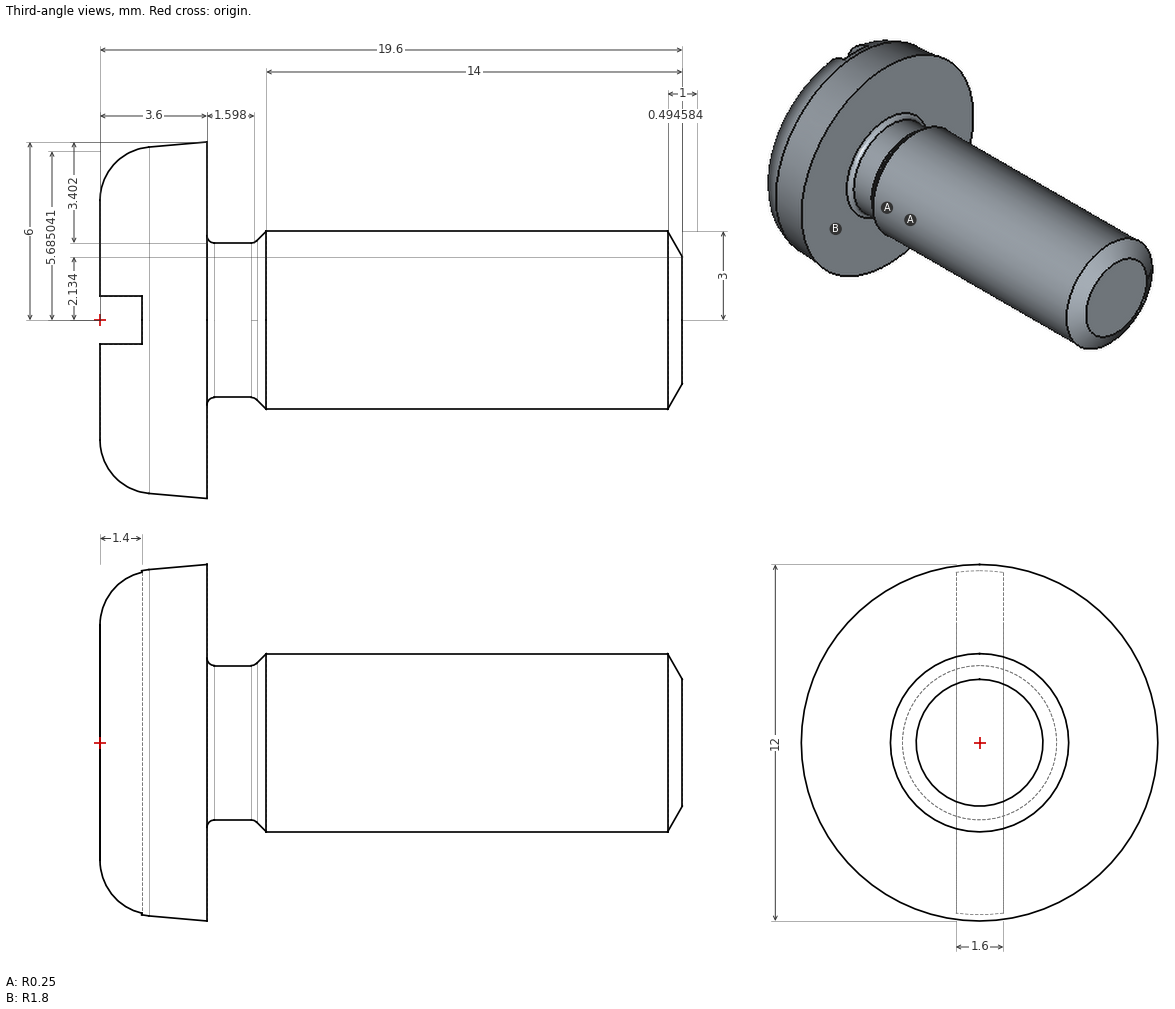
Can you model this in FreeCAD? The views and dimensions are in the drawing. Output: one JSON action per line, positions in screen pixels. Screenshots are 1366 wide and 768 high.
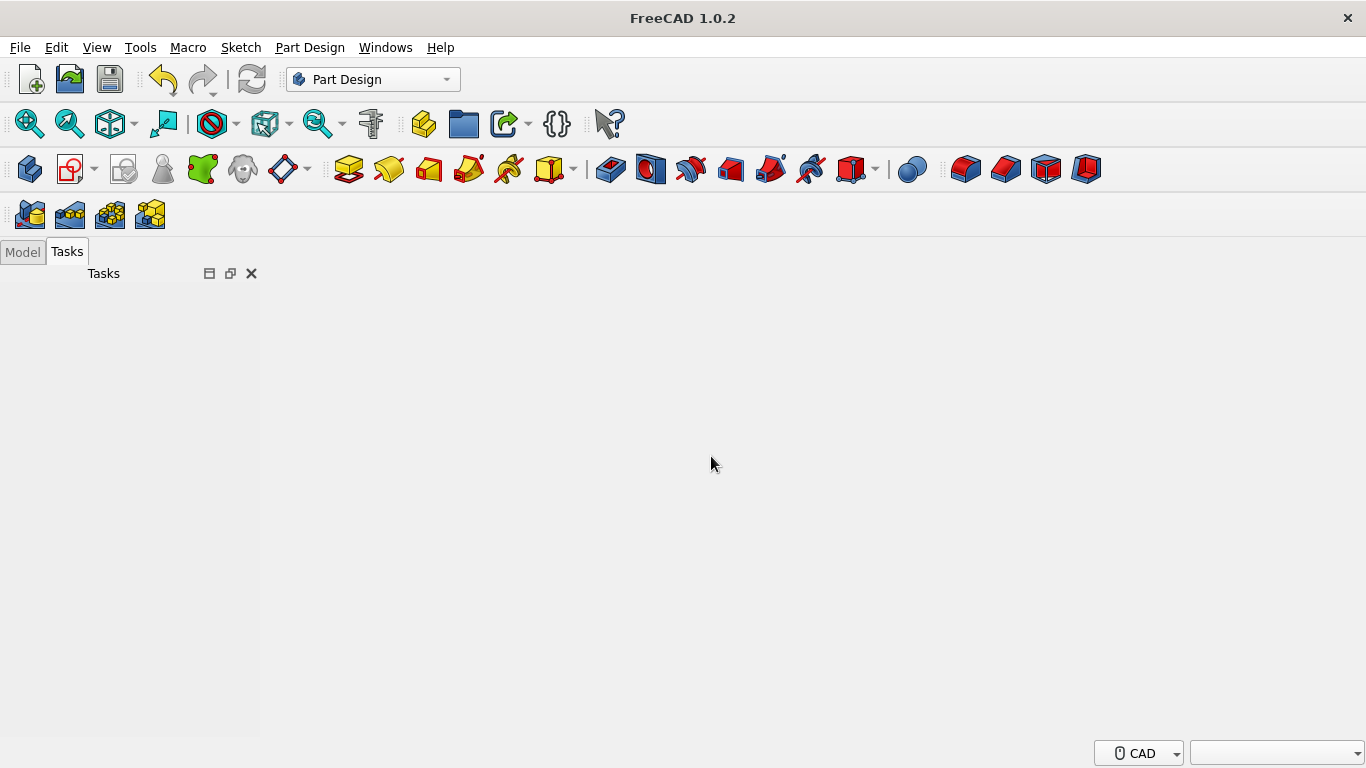
{"action": "left_click", "coordinate": [30, 80]}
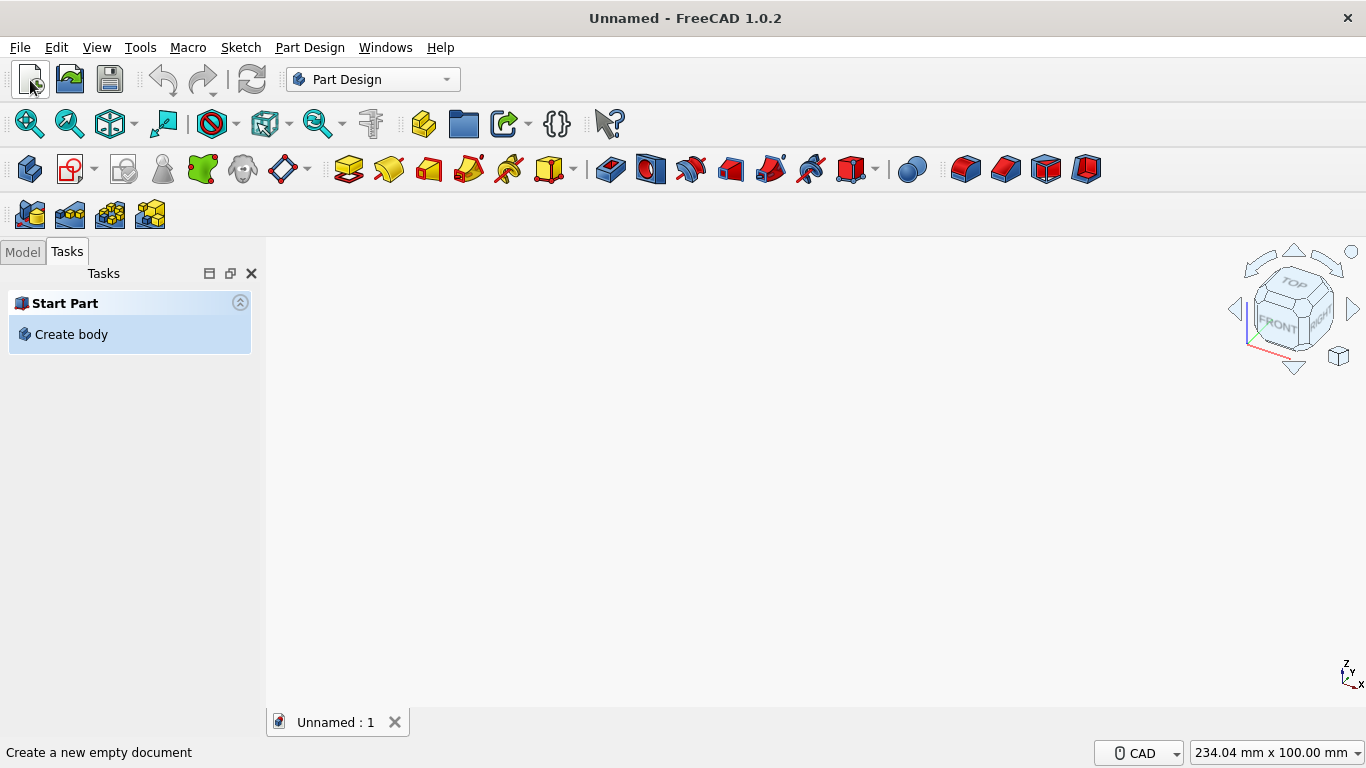
{"action": "left_click", "coordinate": [70, 170]}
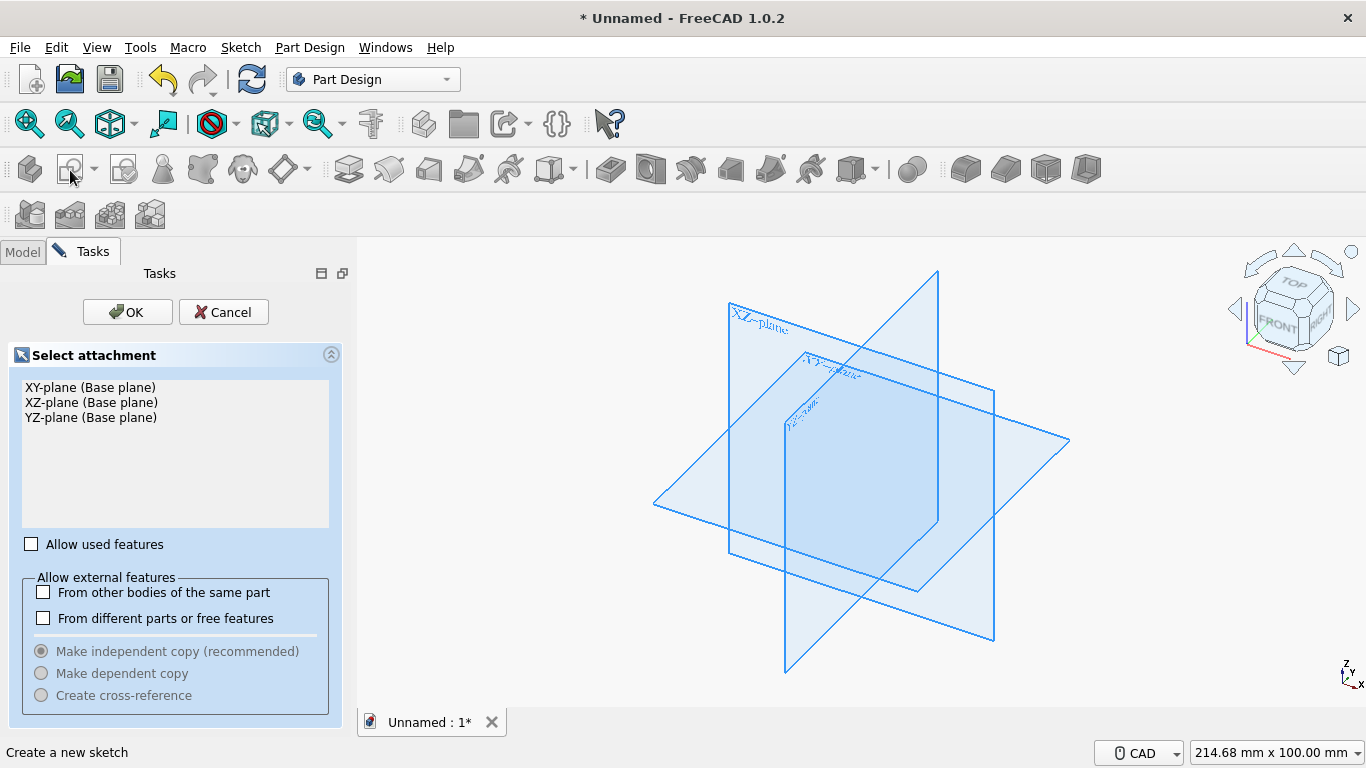
{"action": "left_click", "coordinate": [82, 388]}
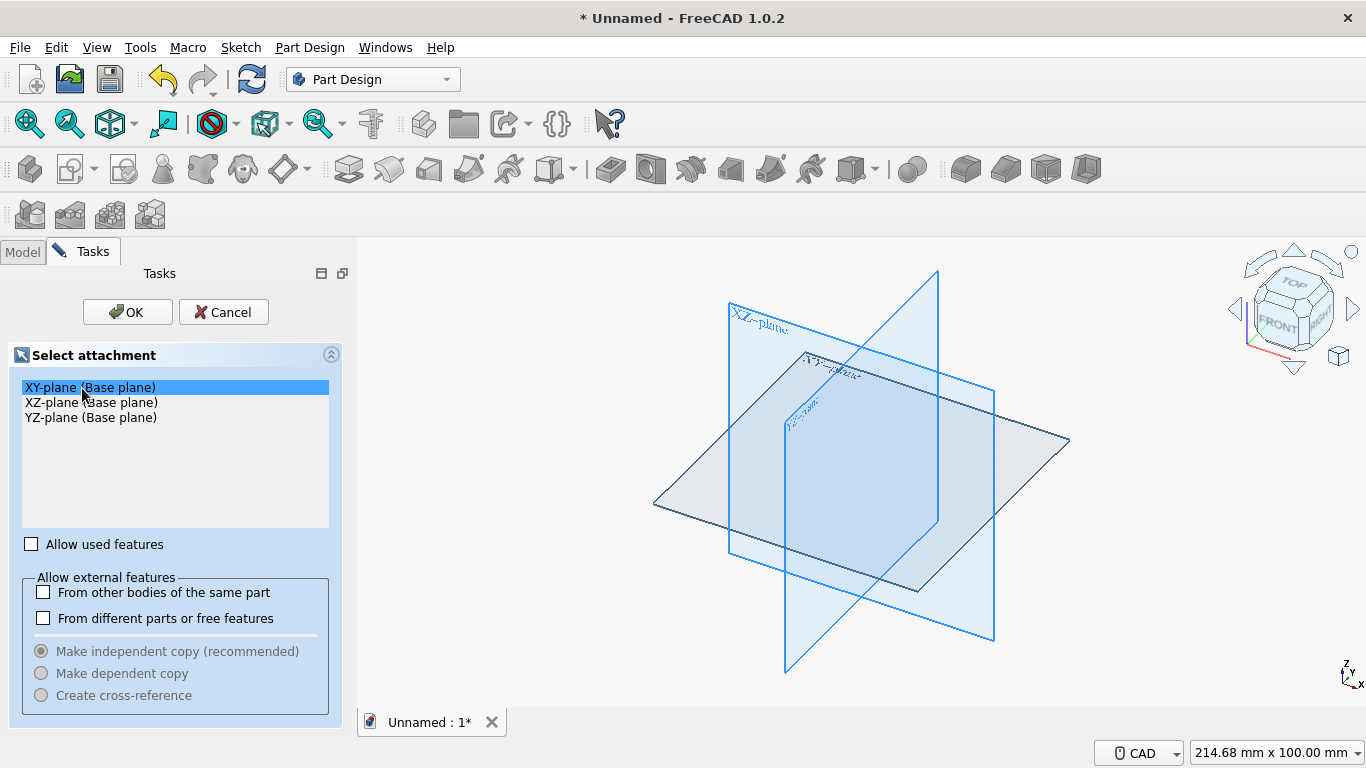
{"action": "left_click", "coordinate": [128, 312]}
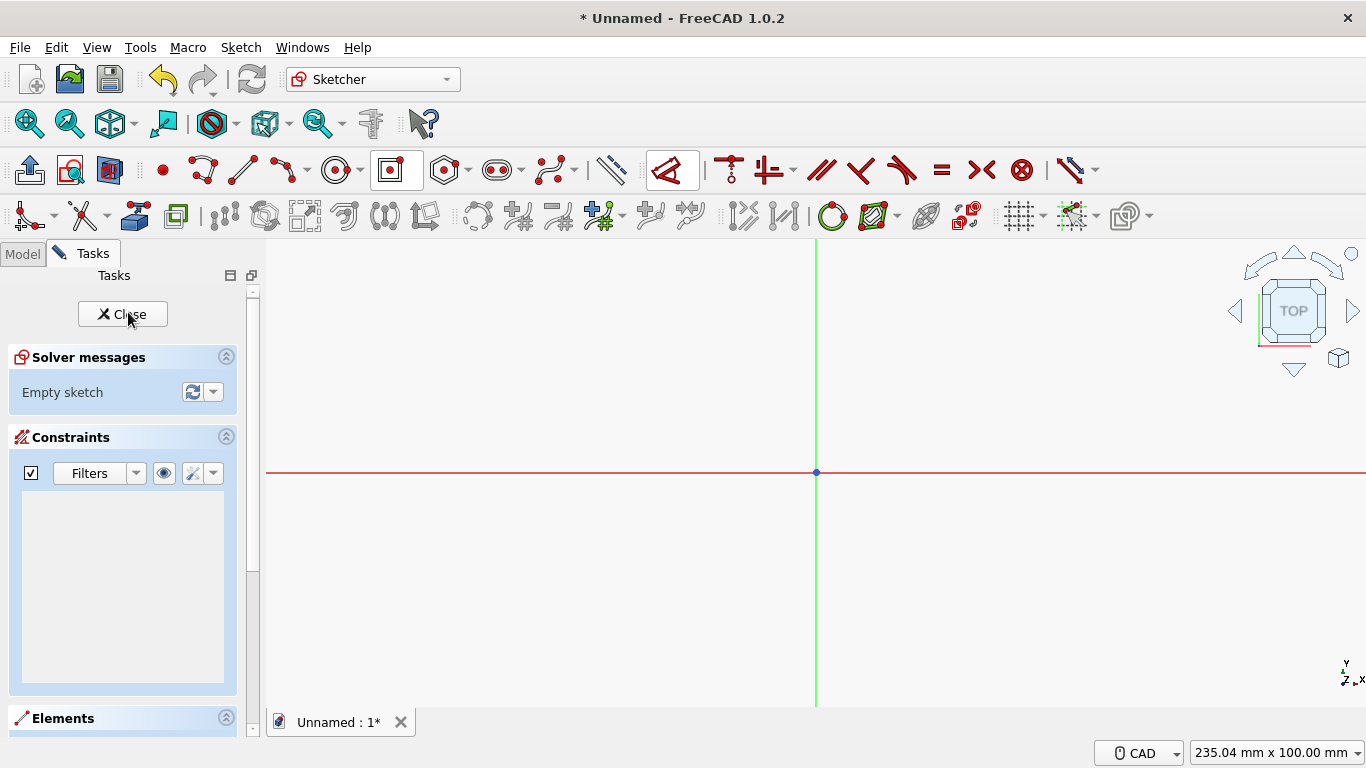
{"action": "scroll", "coordinate": [880, 457], "scroll_direction": "up", "scroll_amount": 10}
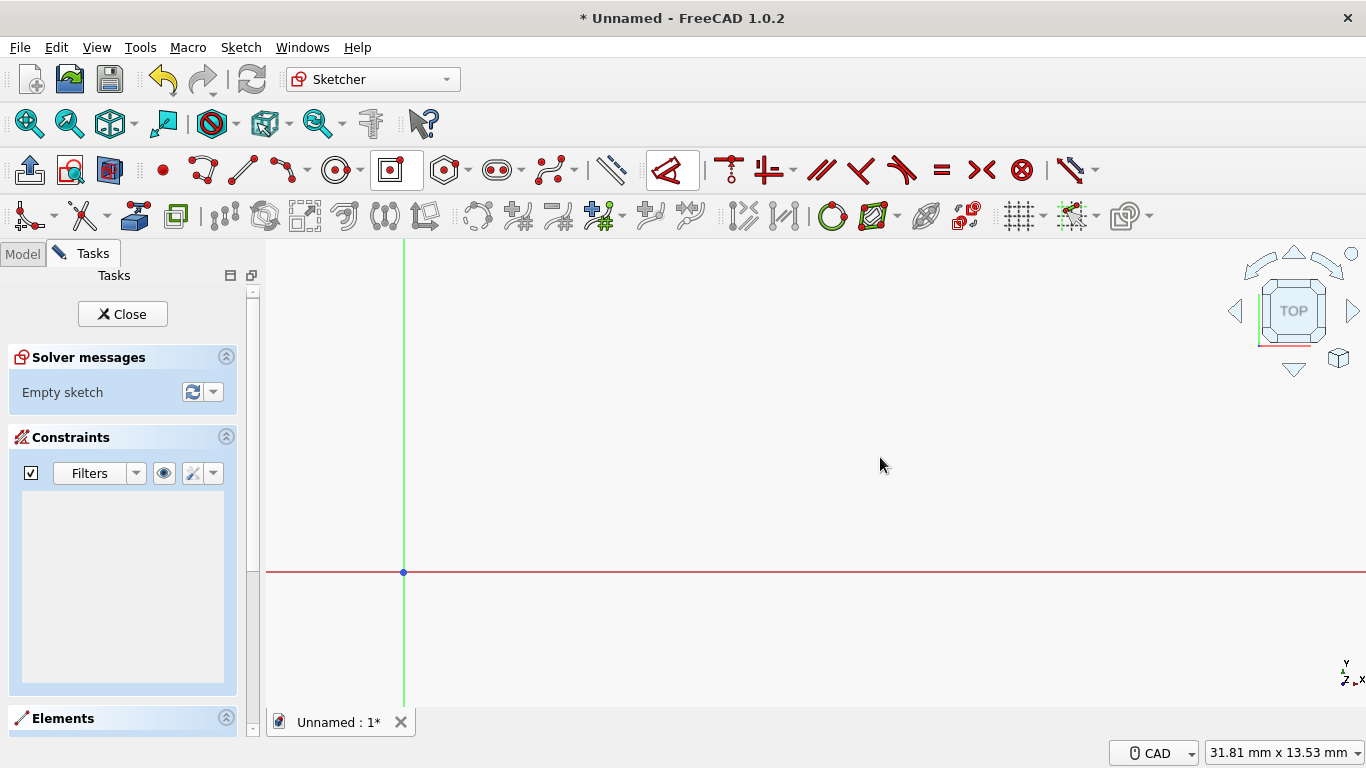
{"action": "left_click", "coordinate": [204, 170]}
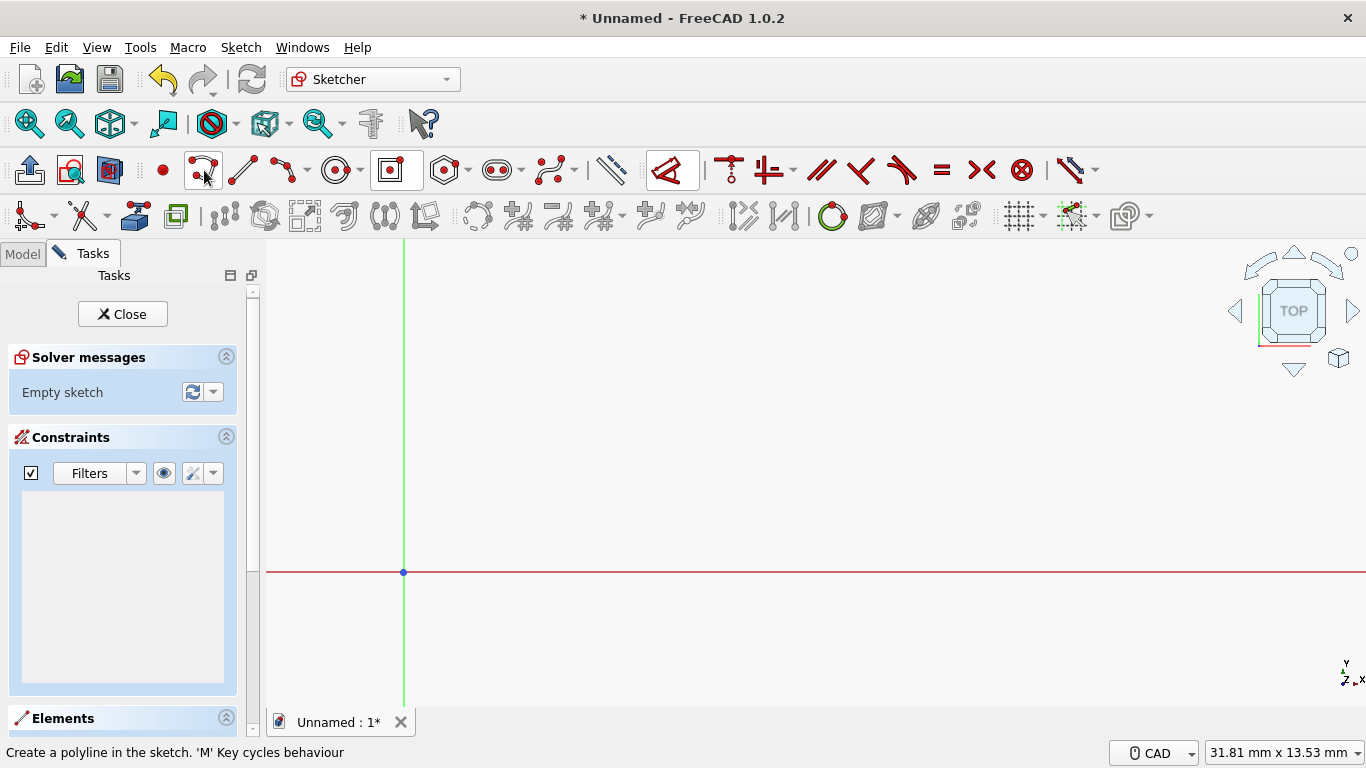
{"action": "left_click", "coordinate": [404, 572]}
{"action": "left_click", "coordinate": [1081, 563]}
{"action": "left_click", "coordinate": [1081, 468]}
{"action": "left_click", "coordinate": [597, 468]}
{"action": "left_click", "coordinate": [583, 482]}
{"action": "left_click", "coordinate": [528, 482]}
{"action": "left_click", "coordinate": [528, 365]}
{"action": "left_click", "coordinate": [413, 376]}
{"action": "left_click", "coordinate": [404, 572]}
{"action": "key", "text": "Escape"}
{"action": "key", "text": "Escape"}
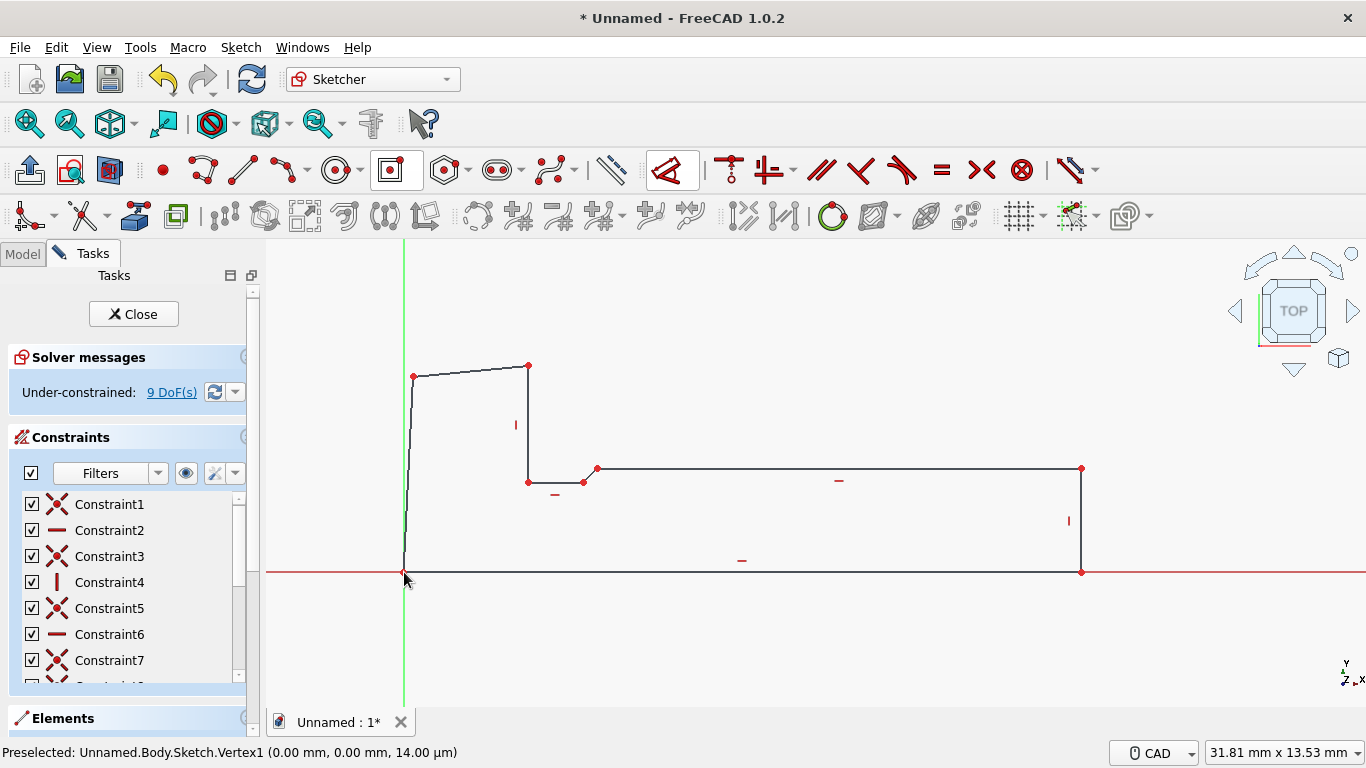
{"action": "left_click", "coordinate": [406, 514]}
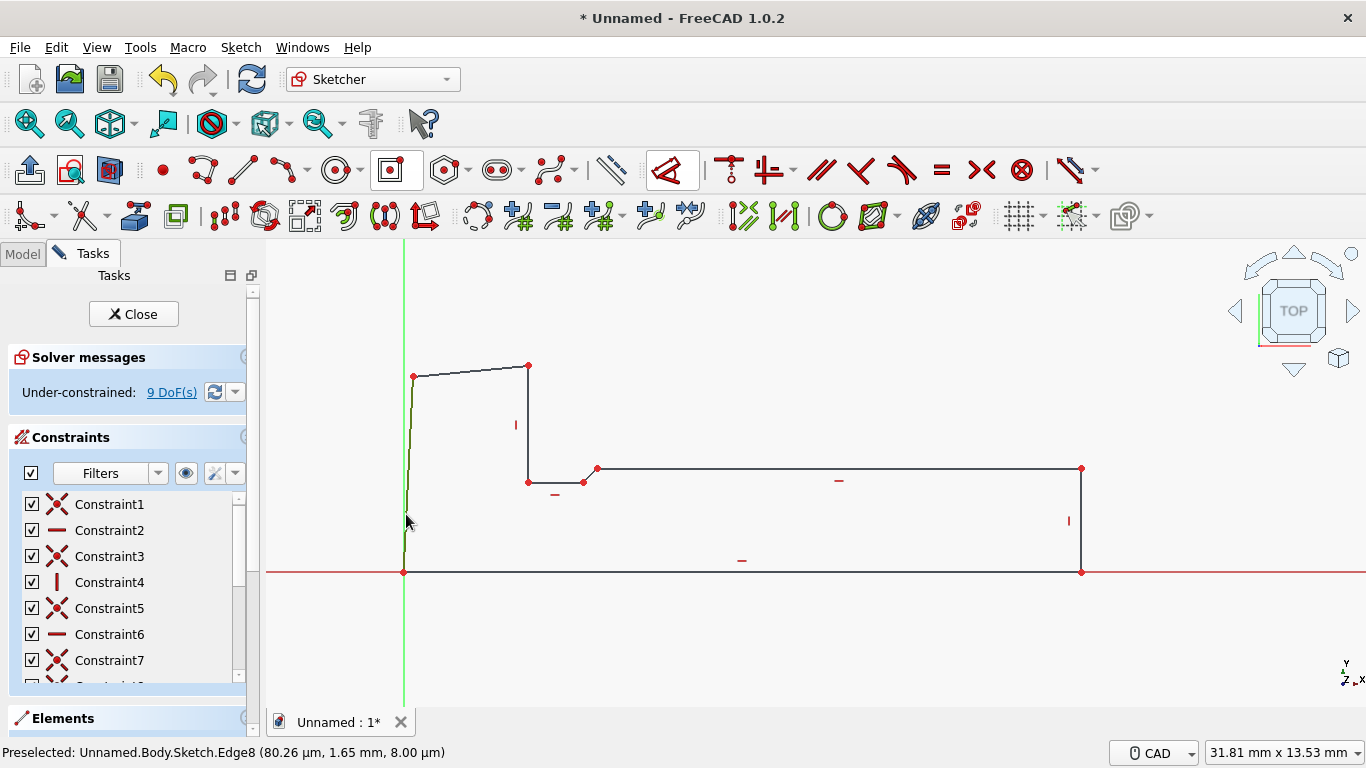
{"action": "left_click", "coordinate": [796, 170]}